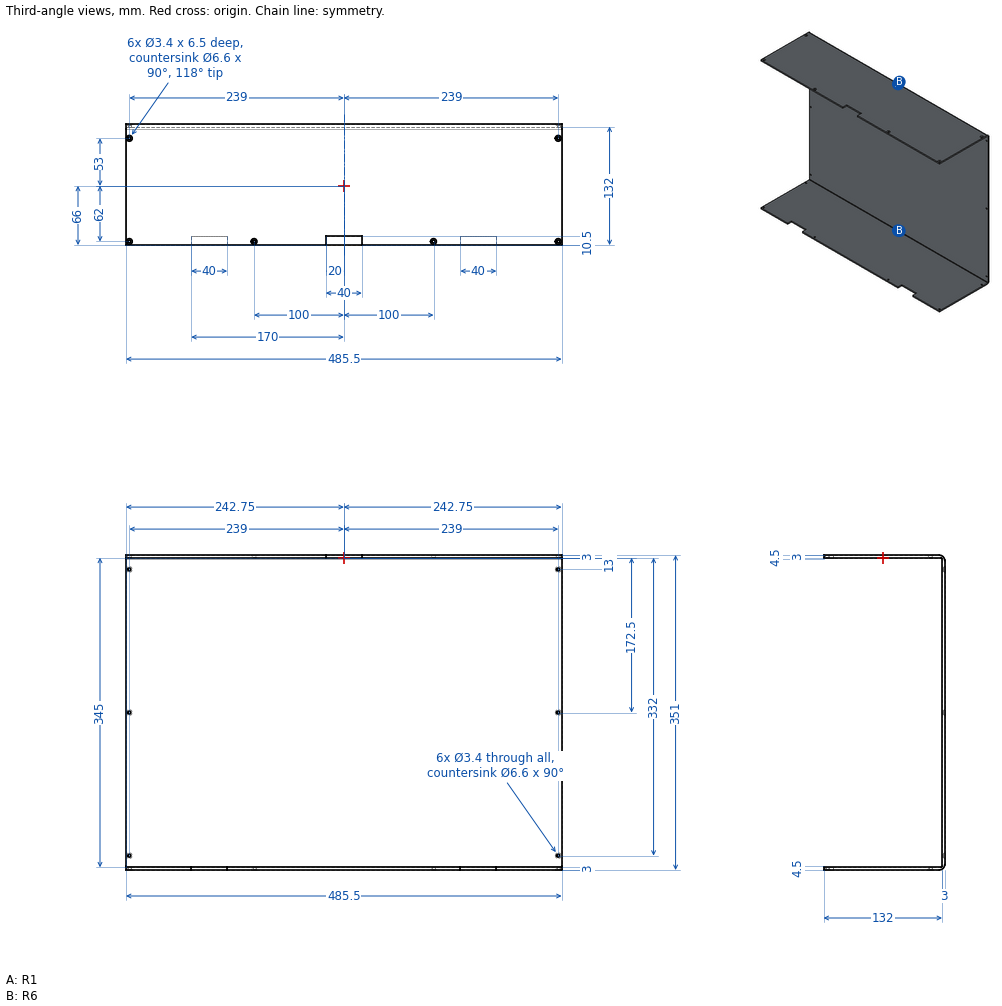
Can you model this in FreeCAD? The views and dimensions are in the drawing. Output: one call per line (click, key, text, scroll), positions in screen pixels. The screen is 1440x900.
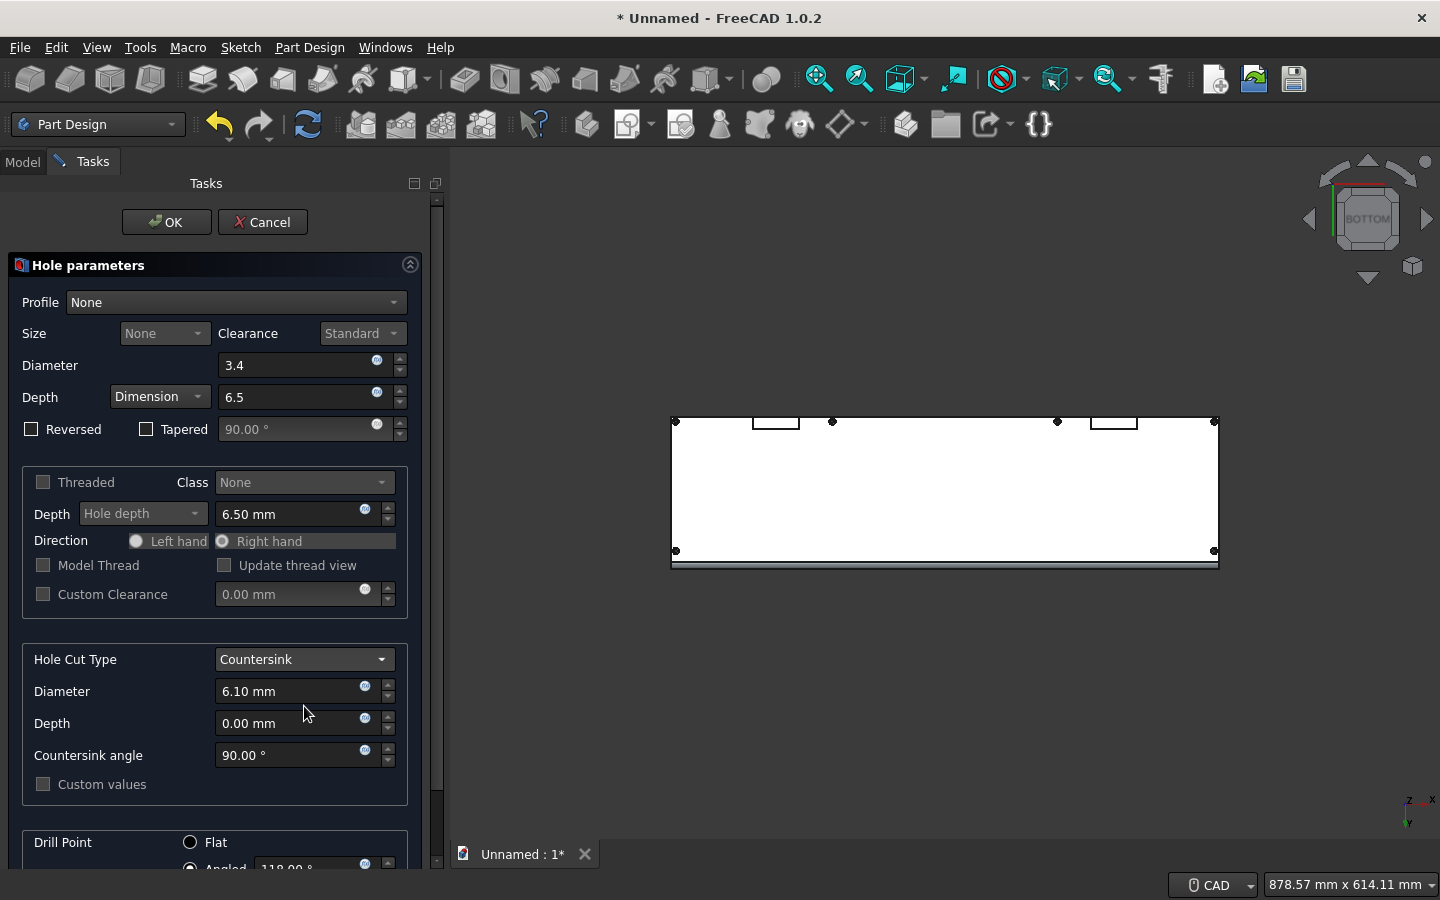
triple_click(298, 691)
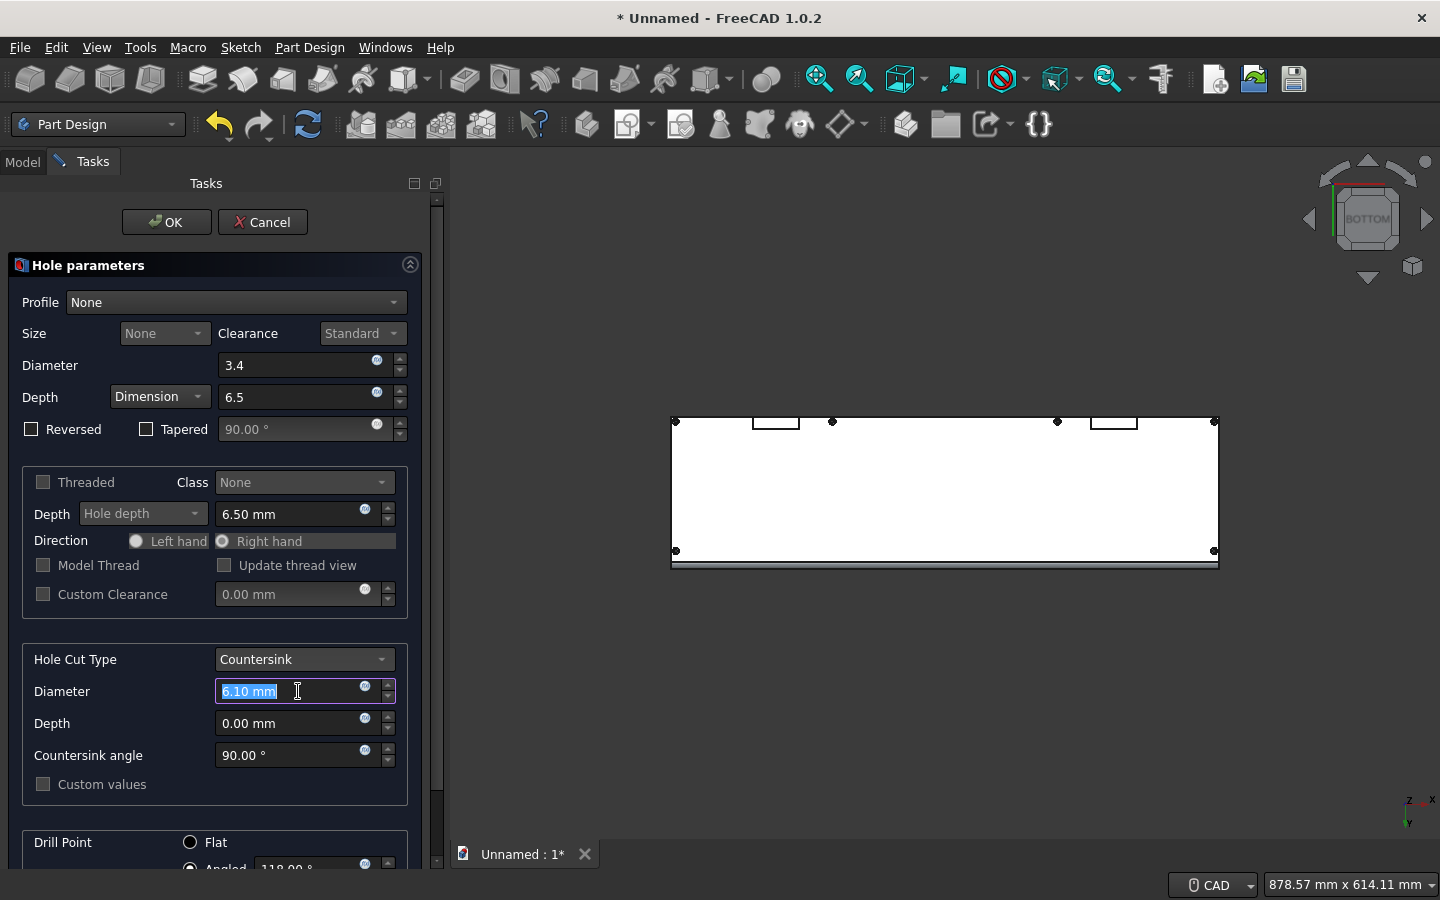
text(6.6)
key(Tab)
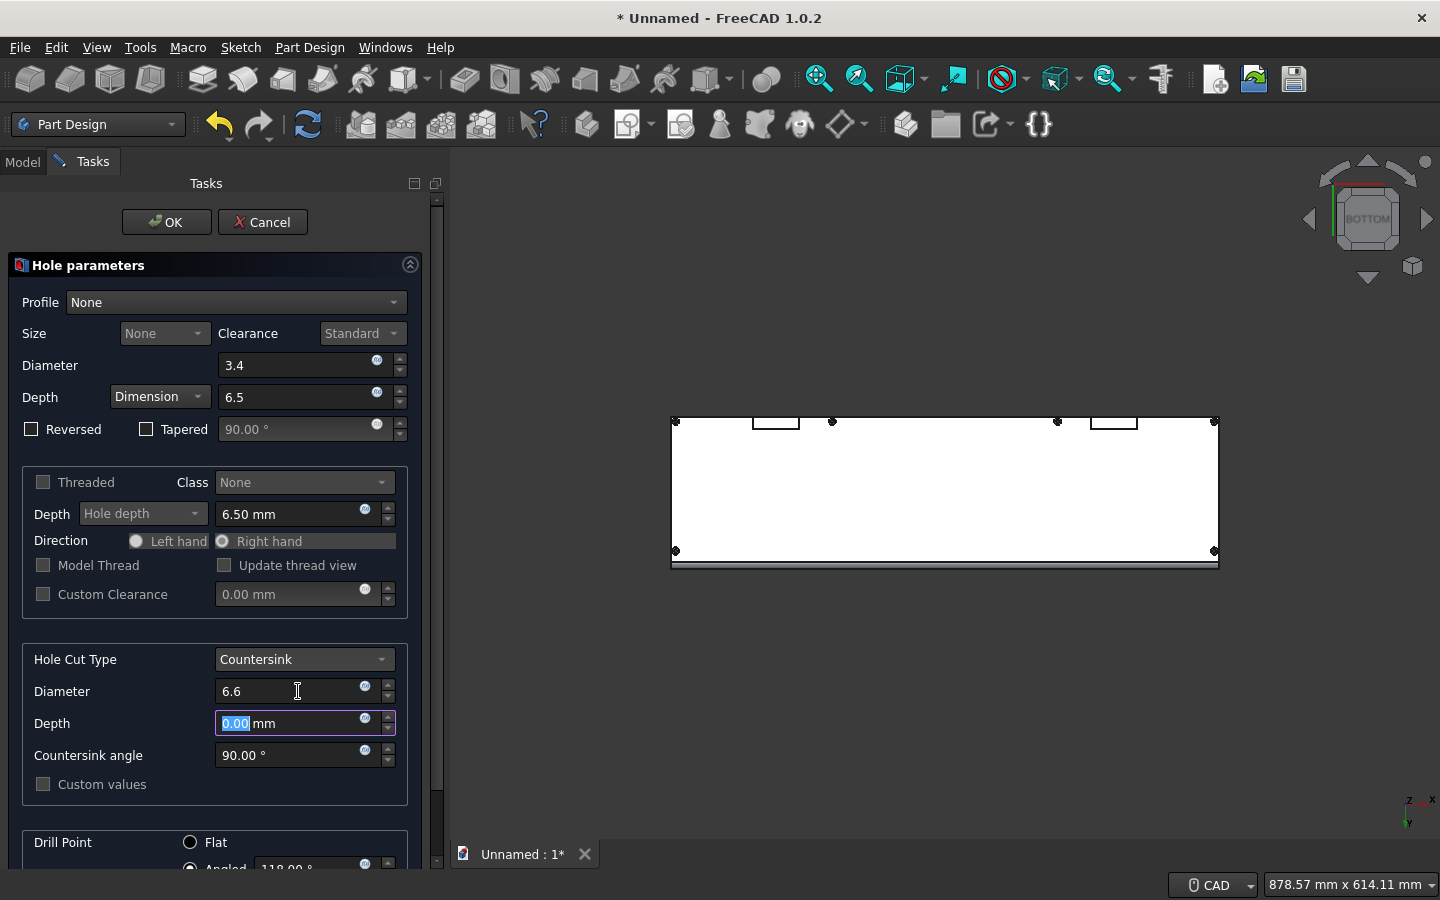
click(167, 222)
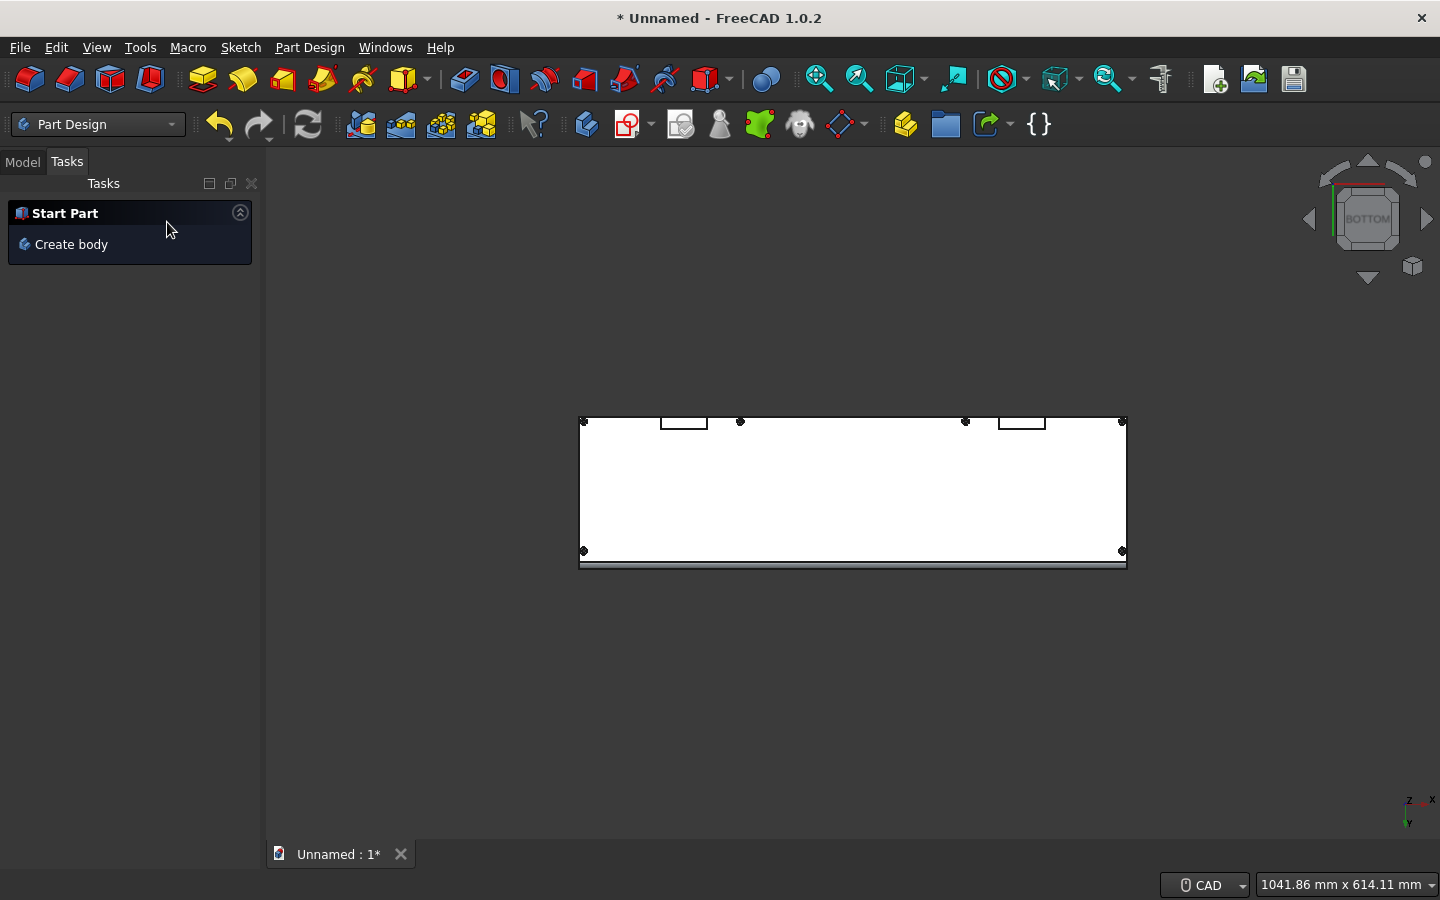
key(0)